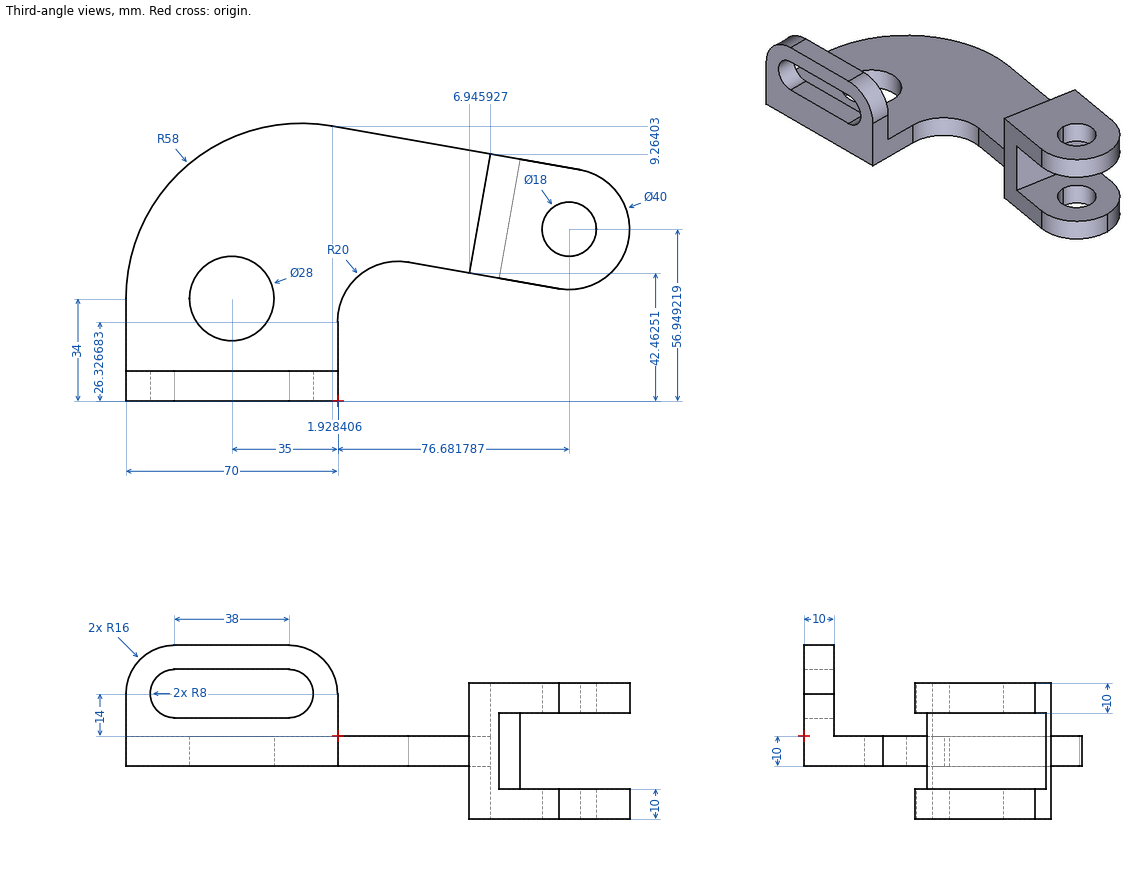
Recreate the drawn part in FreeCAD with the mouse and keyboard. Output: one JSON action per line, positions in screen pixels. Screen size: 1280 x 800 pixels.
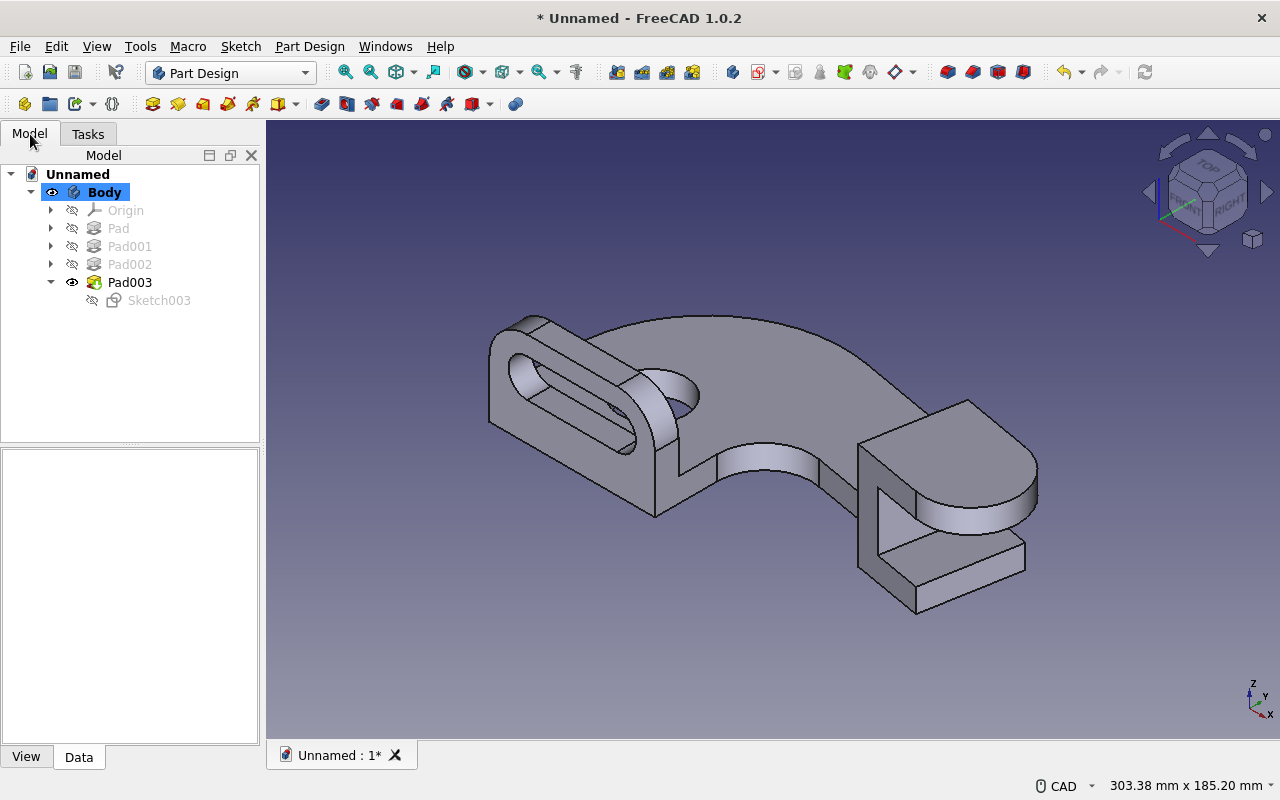
{"action": "left_click", "coordinate": [51, 210]}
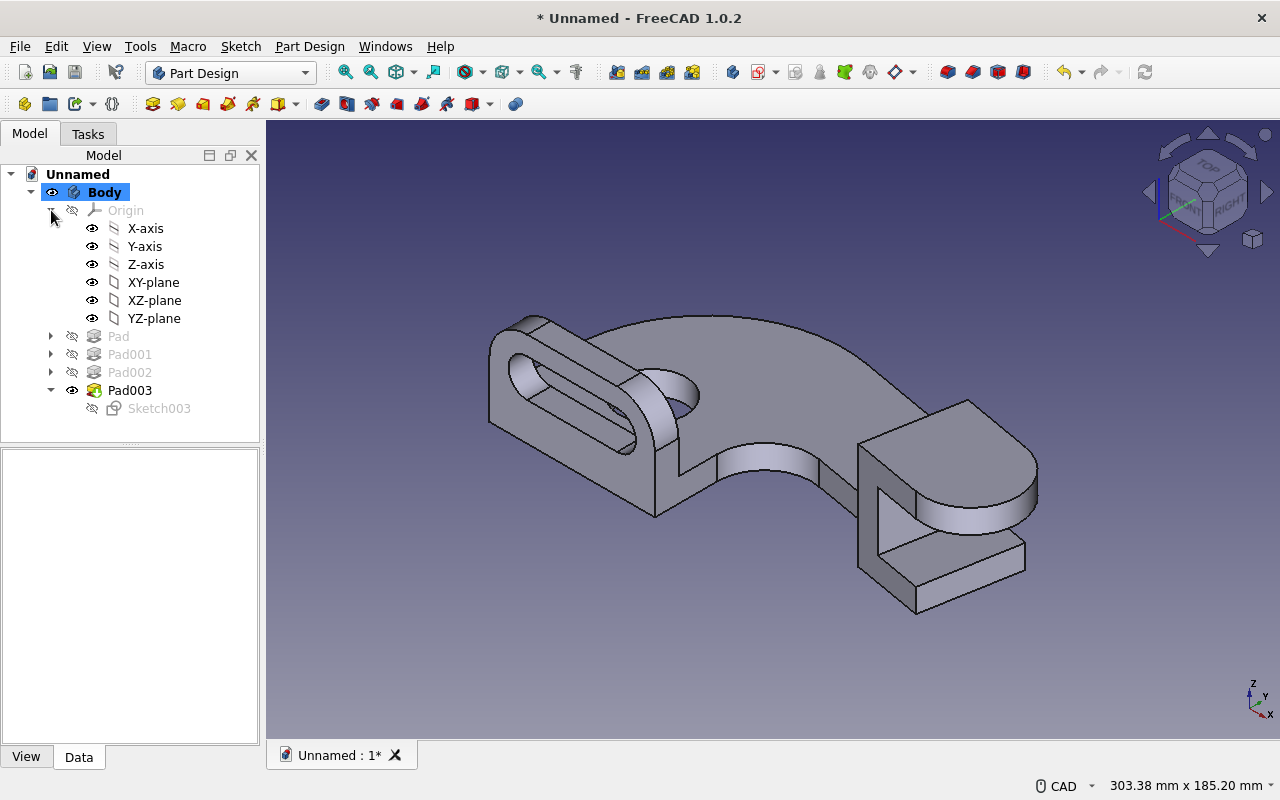
{"action": "left_click", "coordinate": [137, 282]}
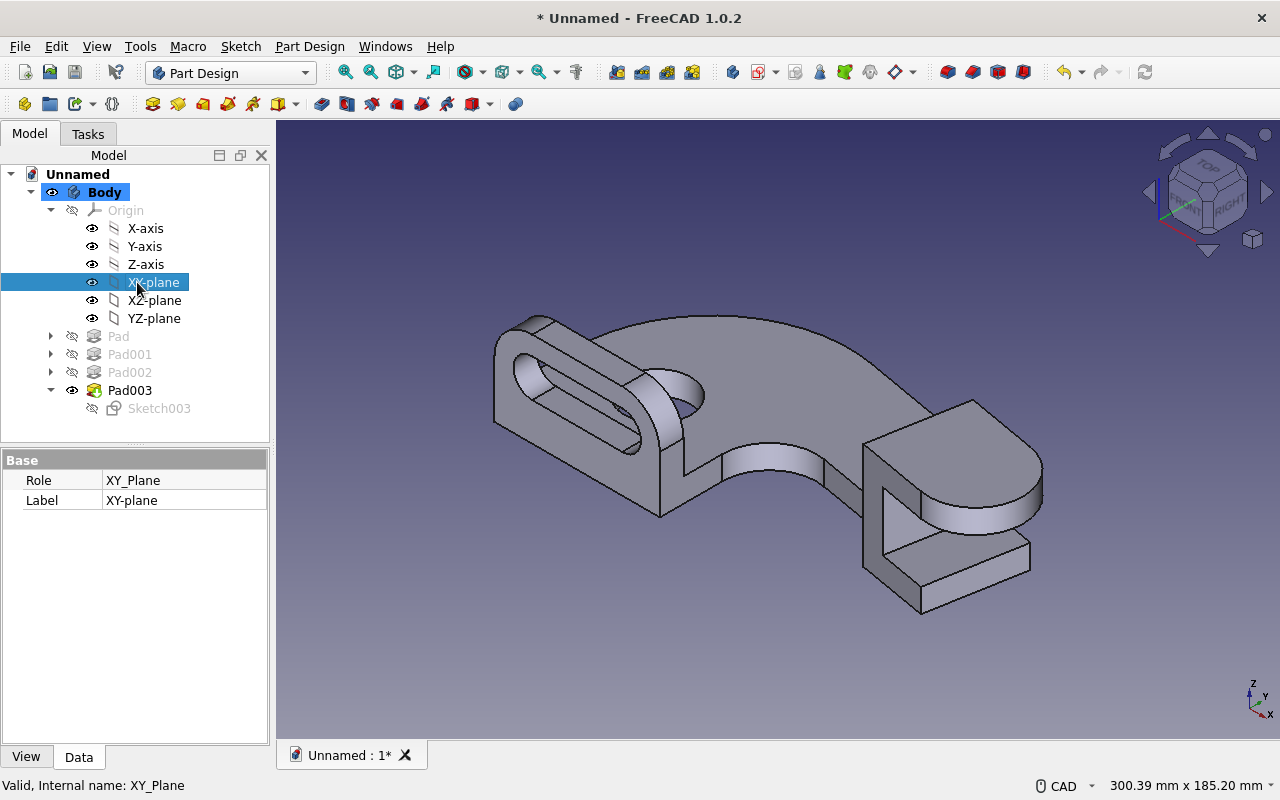
{"action": "left_click", "coordinate": [894, 72]}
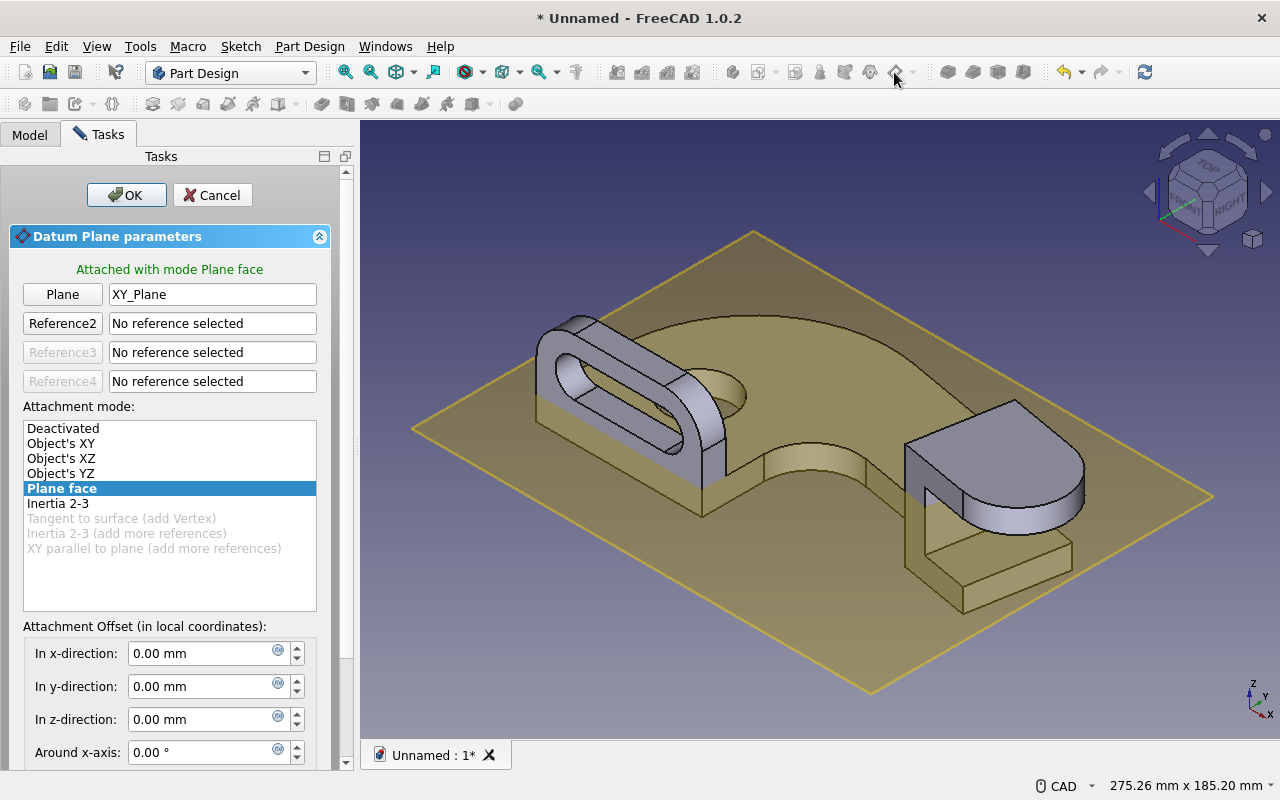
{"action": "triple_click", "coordinate": [210, 720]}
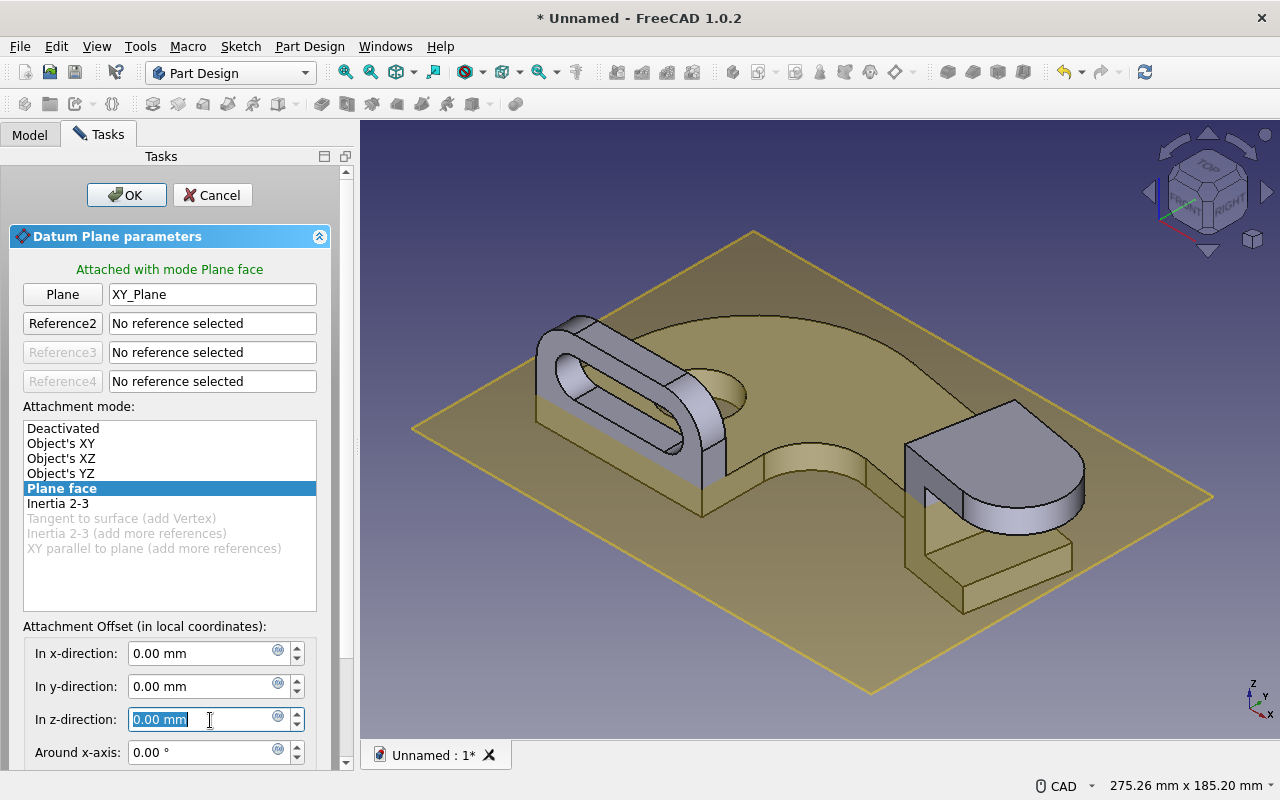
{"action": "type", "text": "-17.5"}
{"action": "key", "text": "Tab"}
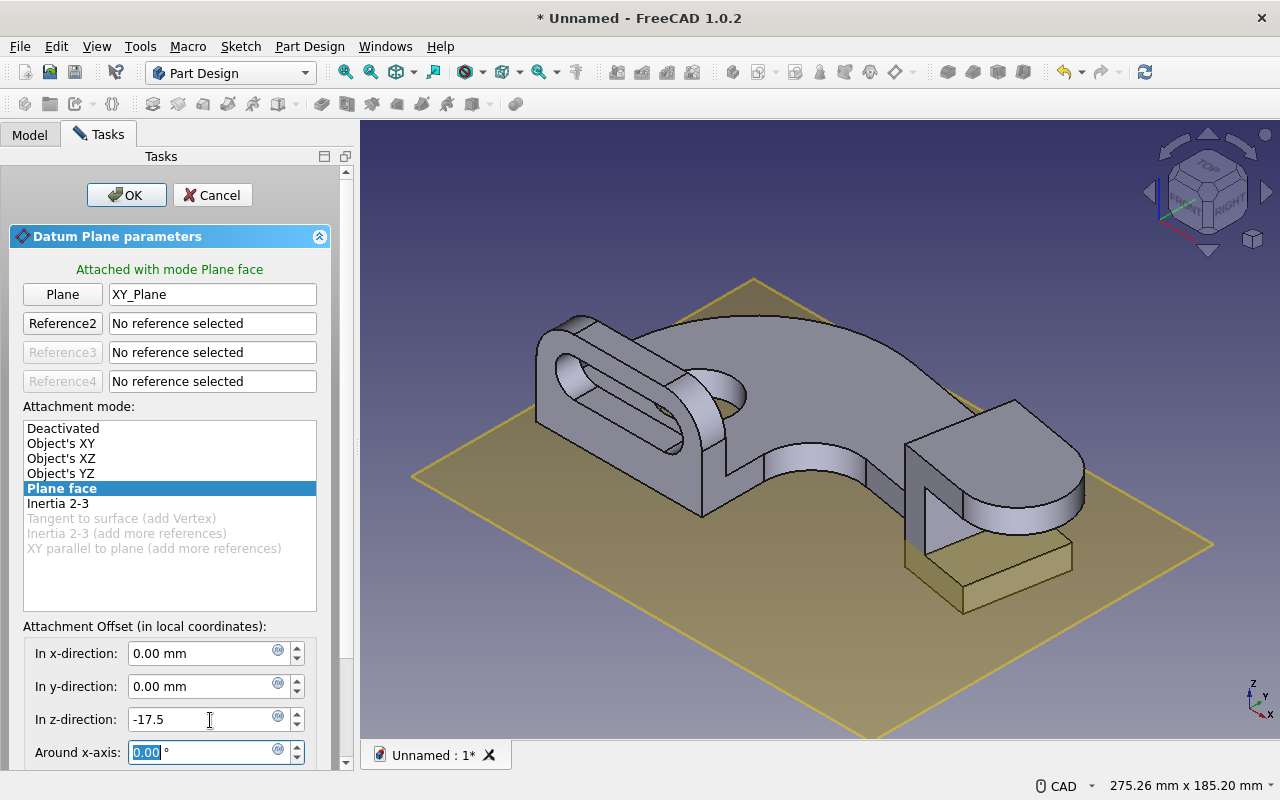
{"action": "left_click", "coordinate": [127, 195]}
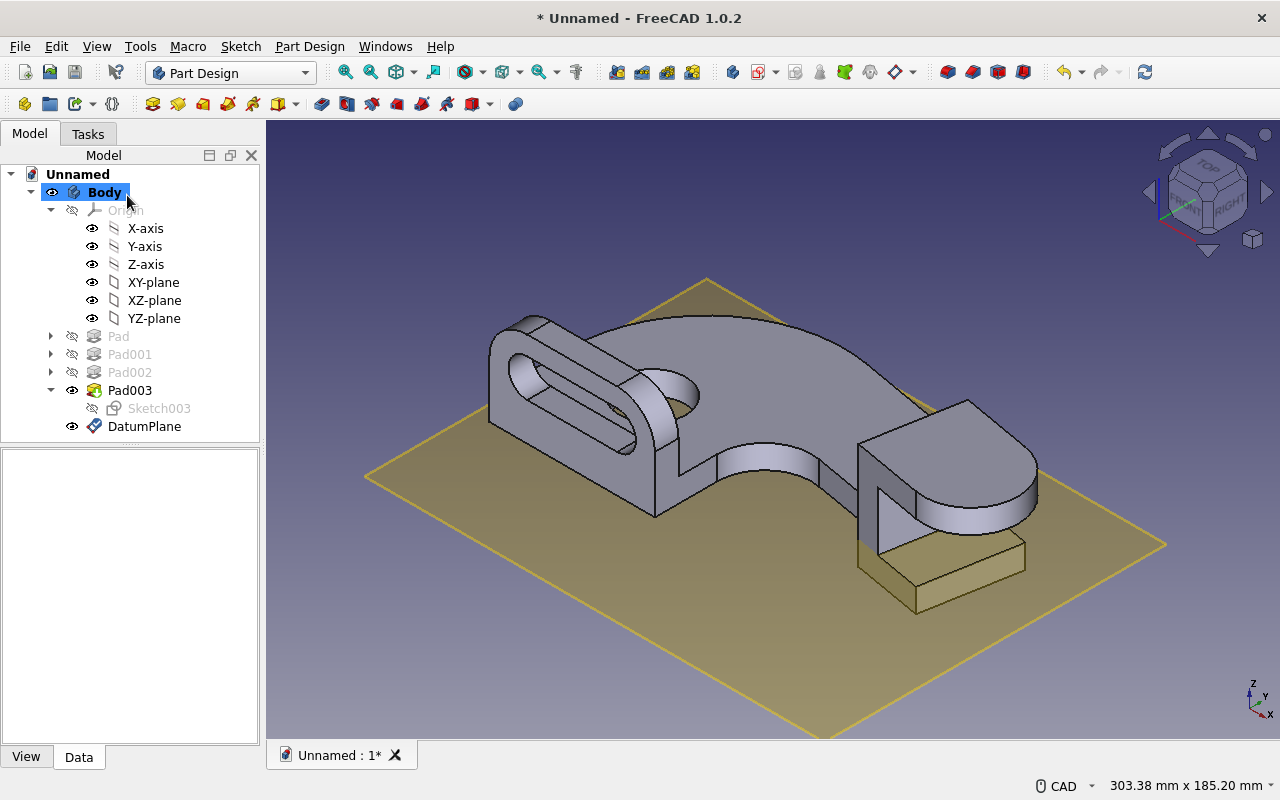
{"action": "left_click", "coordinate": [117, 426]}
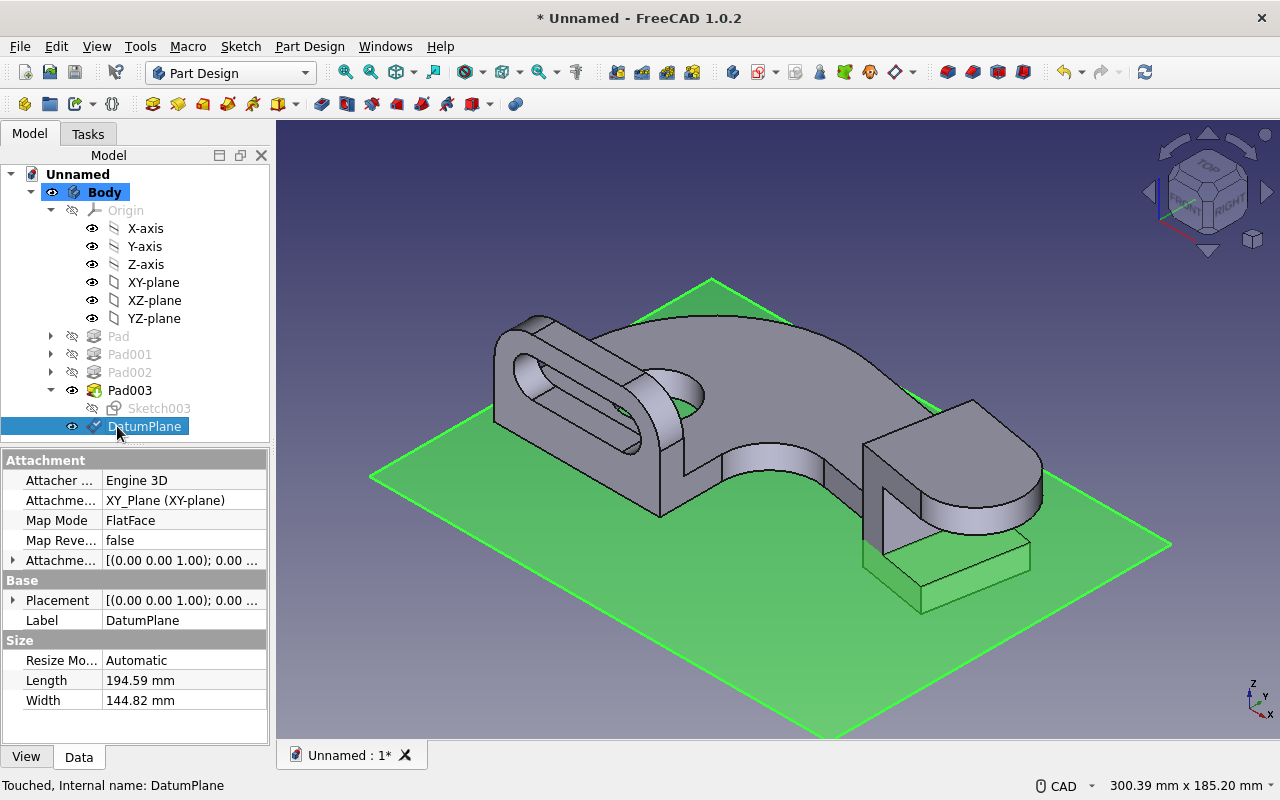
{"action": "left_click", "coordinate": [758, 72]}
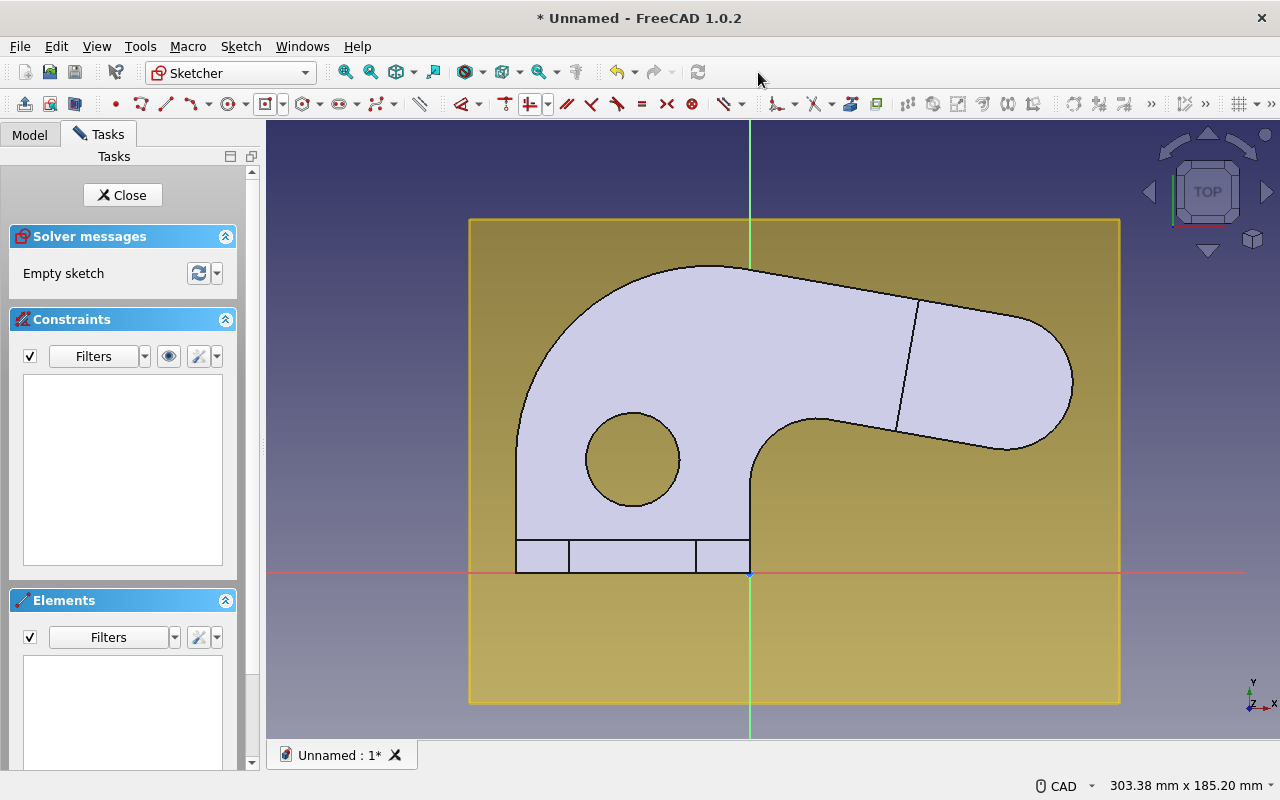
{"action": "left_click", "coordinate": [75, 104]}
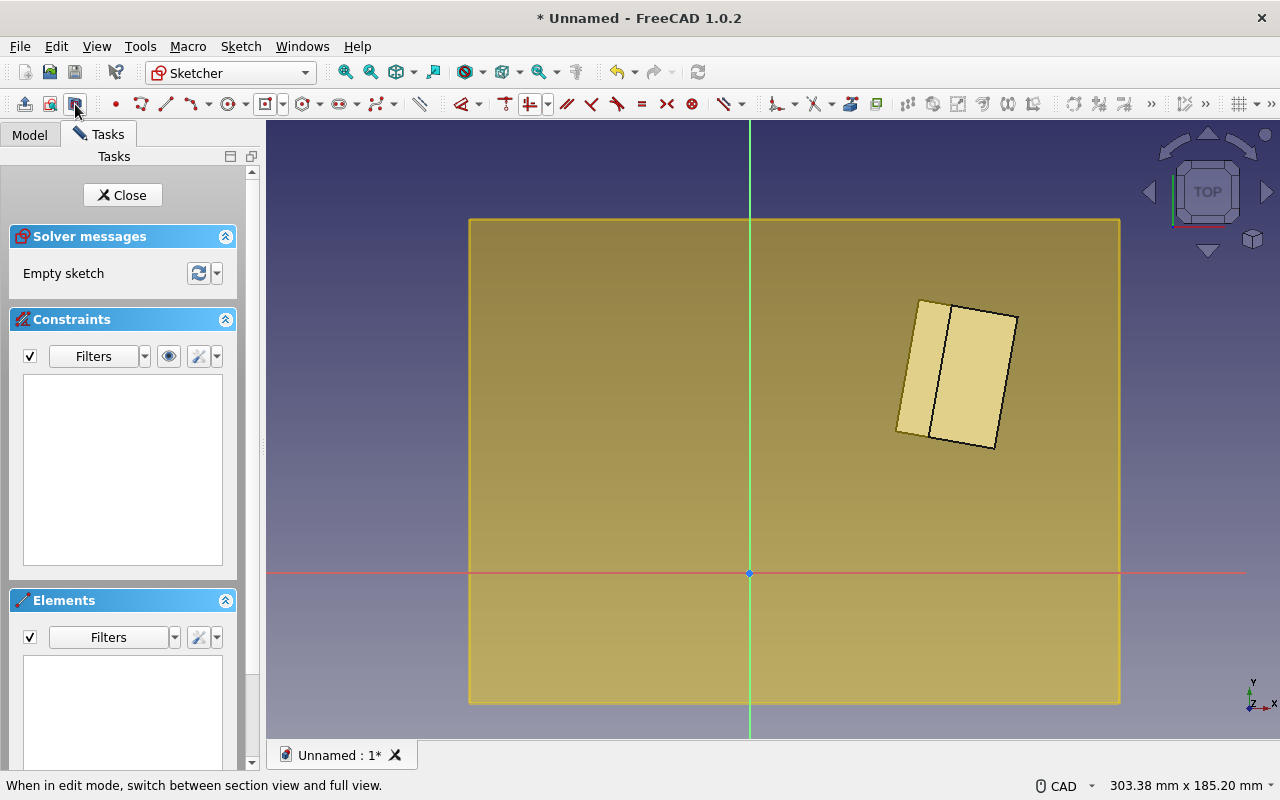
{"action": "scroll", "coordinate": [1115, 475], "scroll_direction": "up", "scroll_amount": 2}